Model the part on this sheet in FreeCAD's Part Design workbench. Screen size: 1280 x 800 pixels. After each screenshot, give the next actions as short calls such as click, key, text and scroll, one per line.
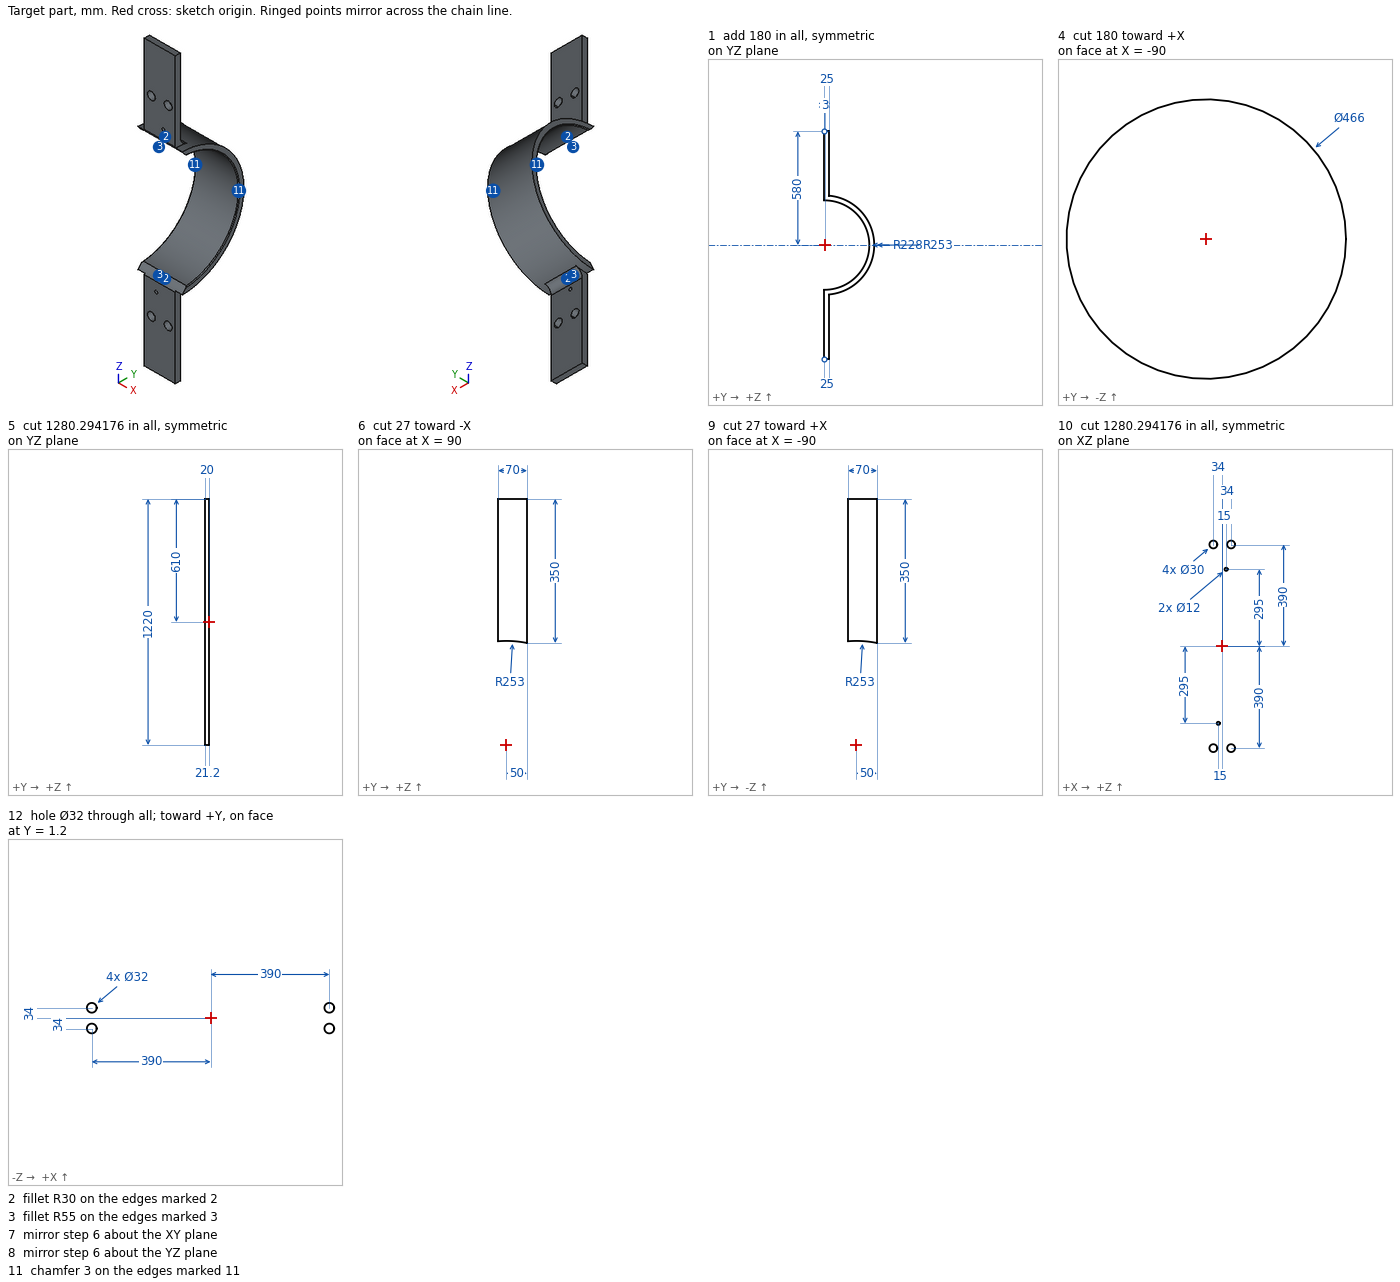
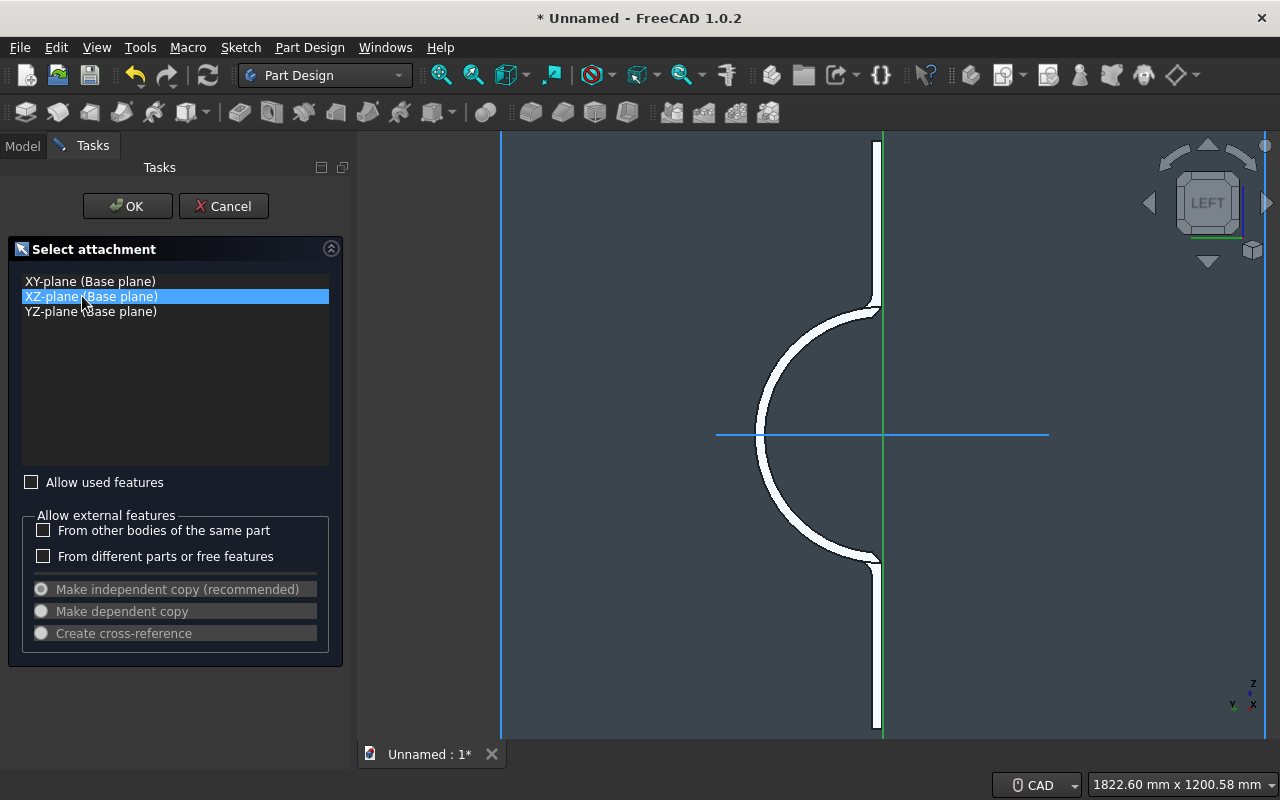
click(128, 206)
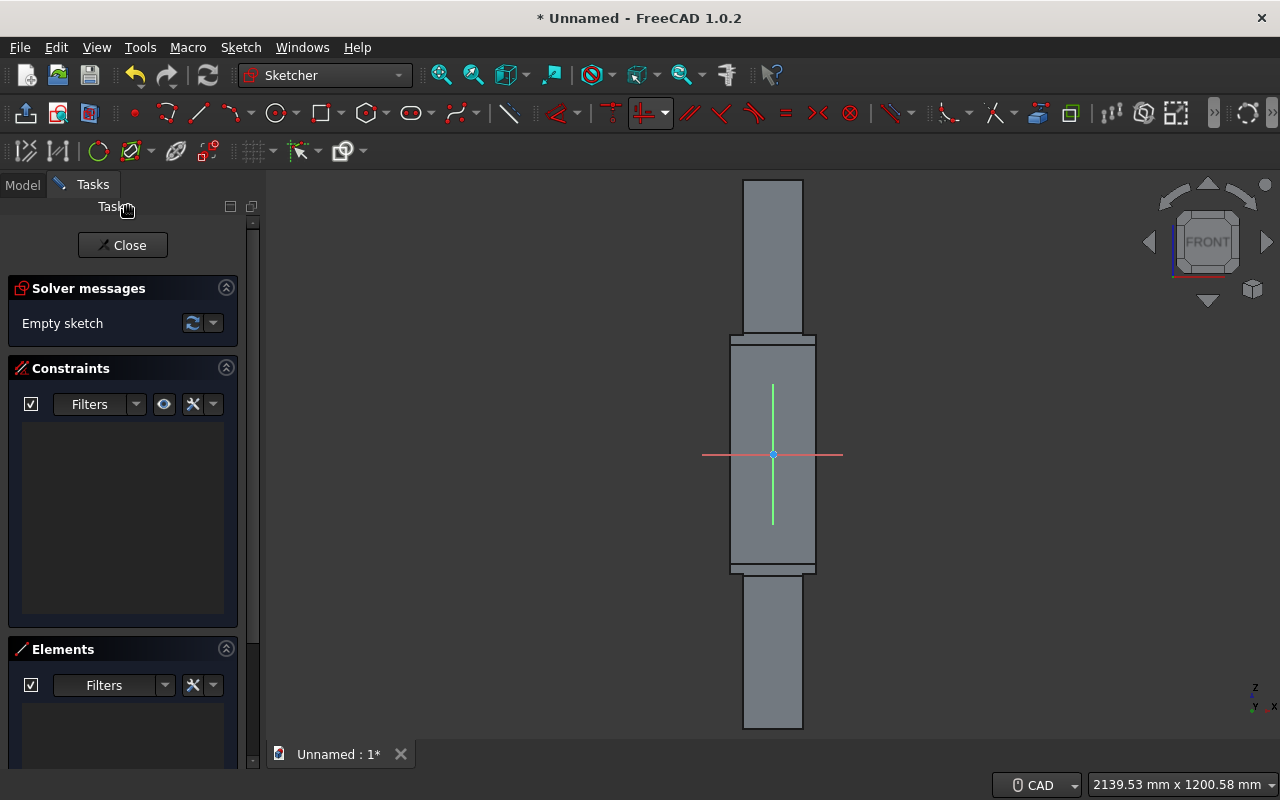
click(276, 114)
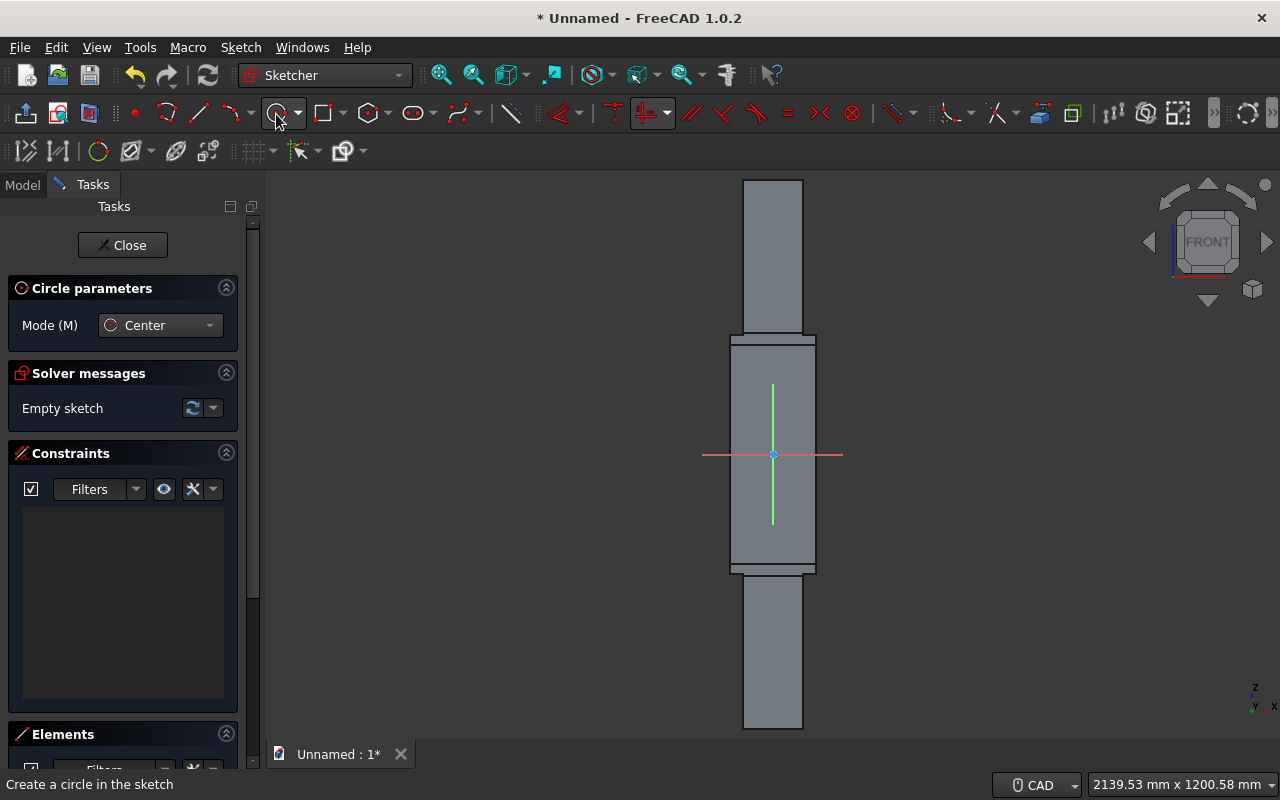
scroll(789, 270, up, 6)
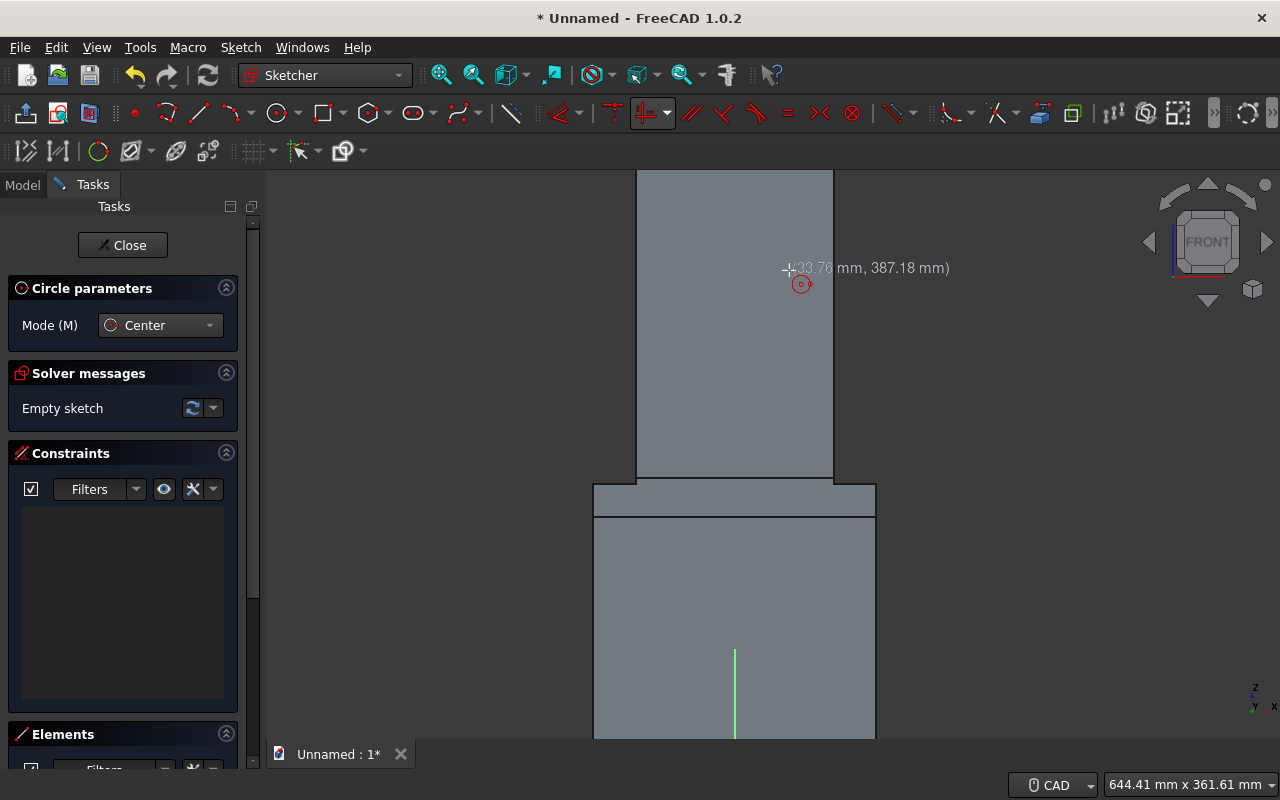
click(788, 268)
move(805, 252)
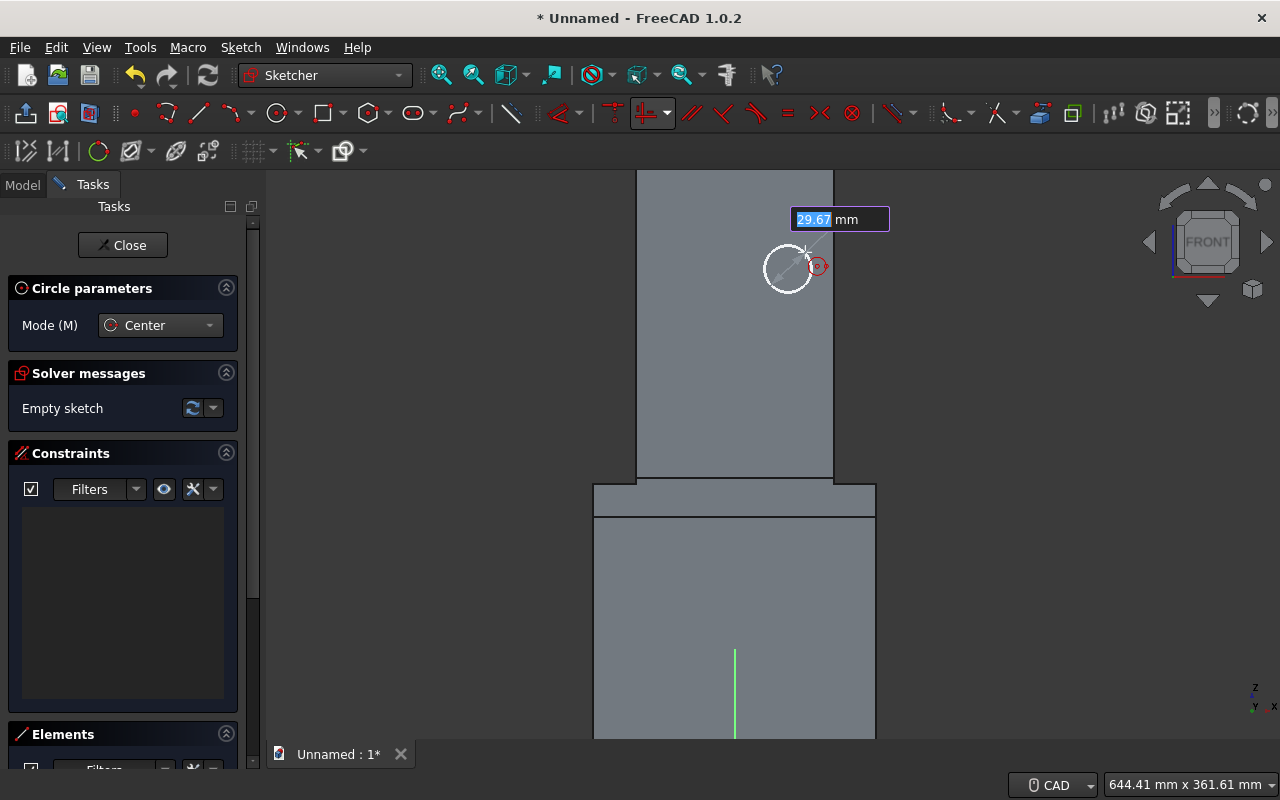
text(30)
key(Return)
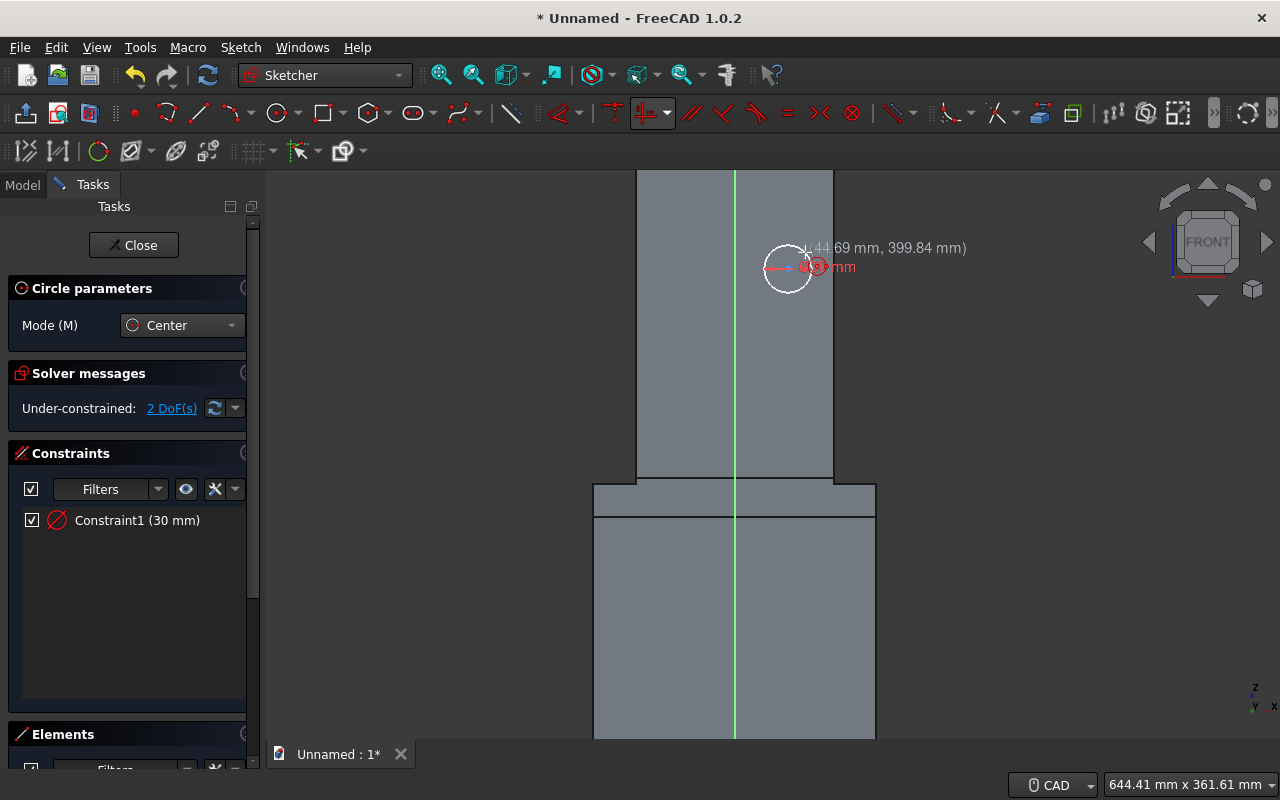
scroll(691, 270, down, 6)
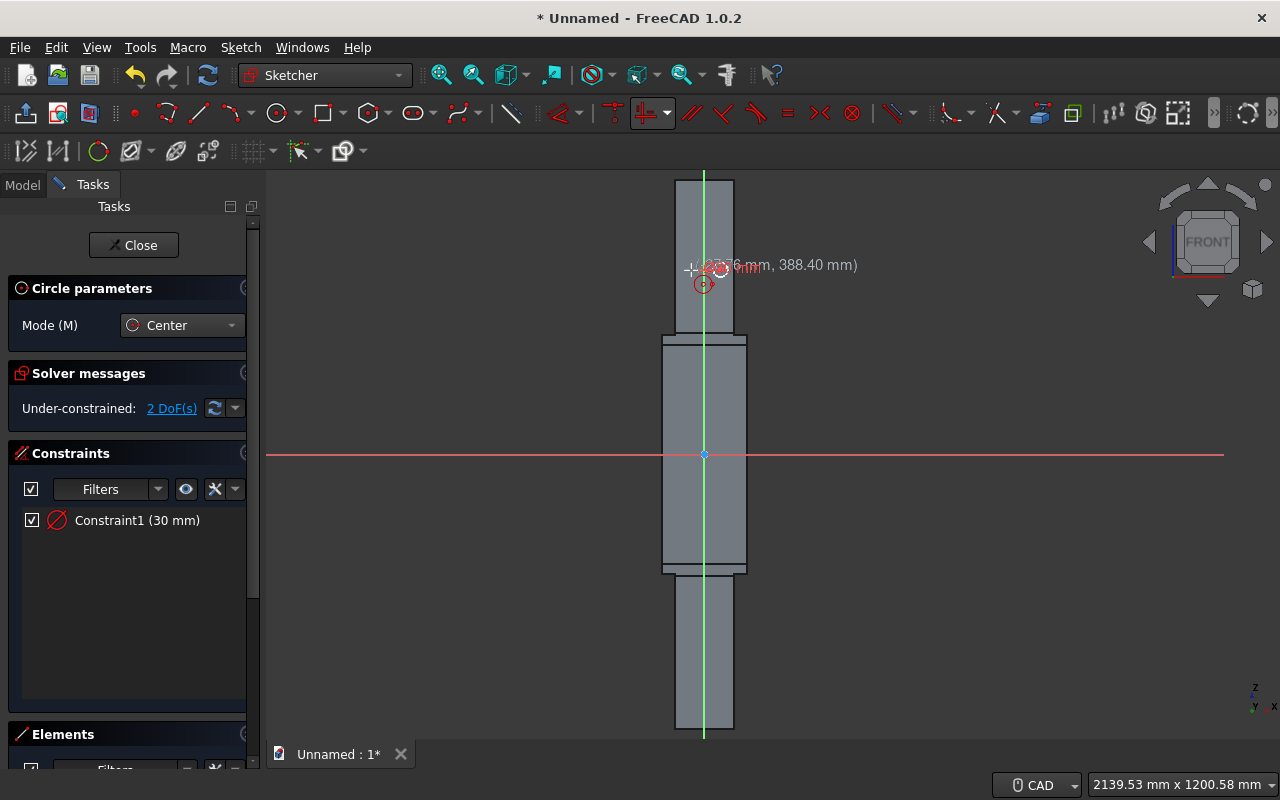
scroll(721, 639, up, 6)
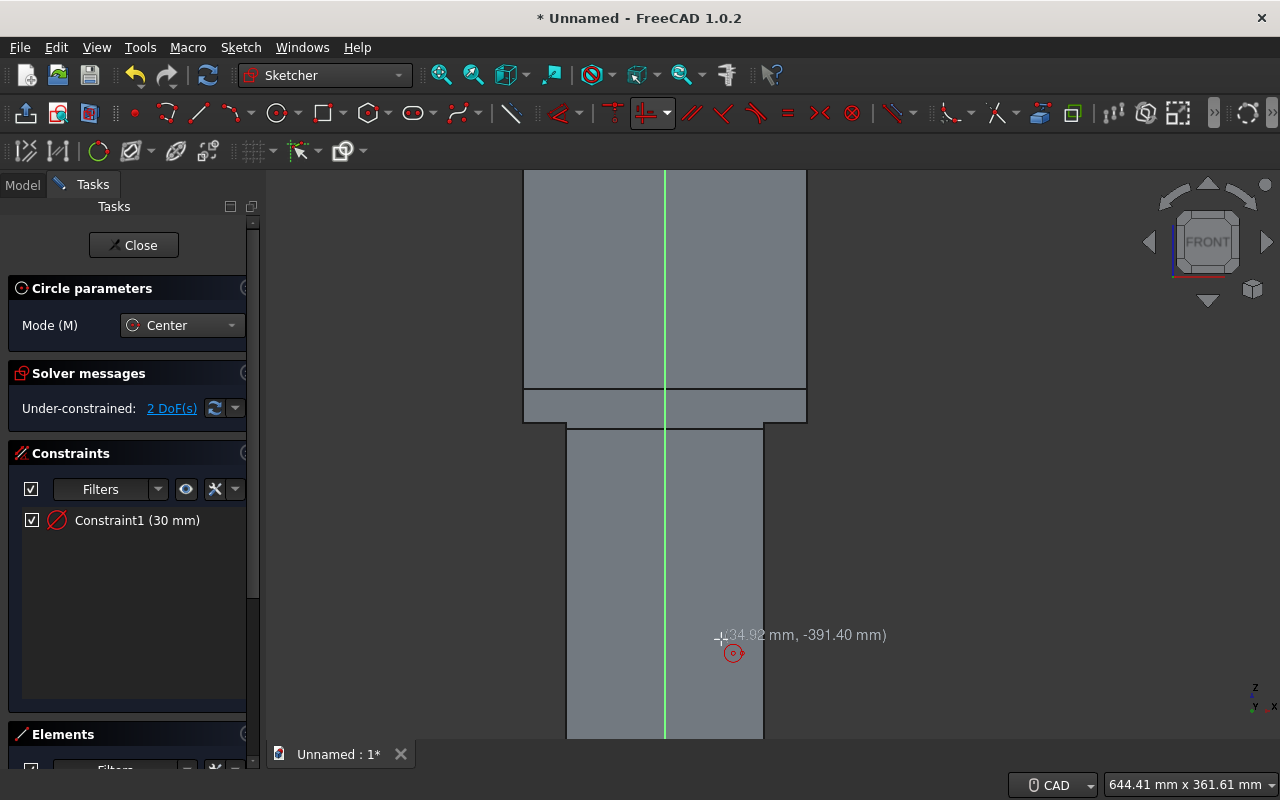
click(719, 638)
move(735, 622)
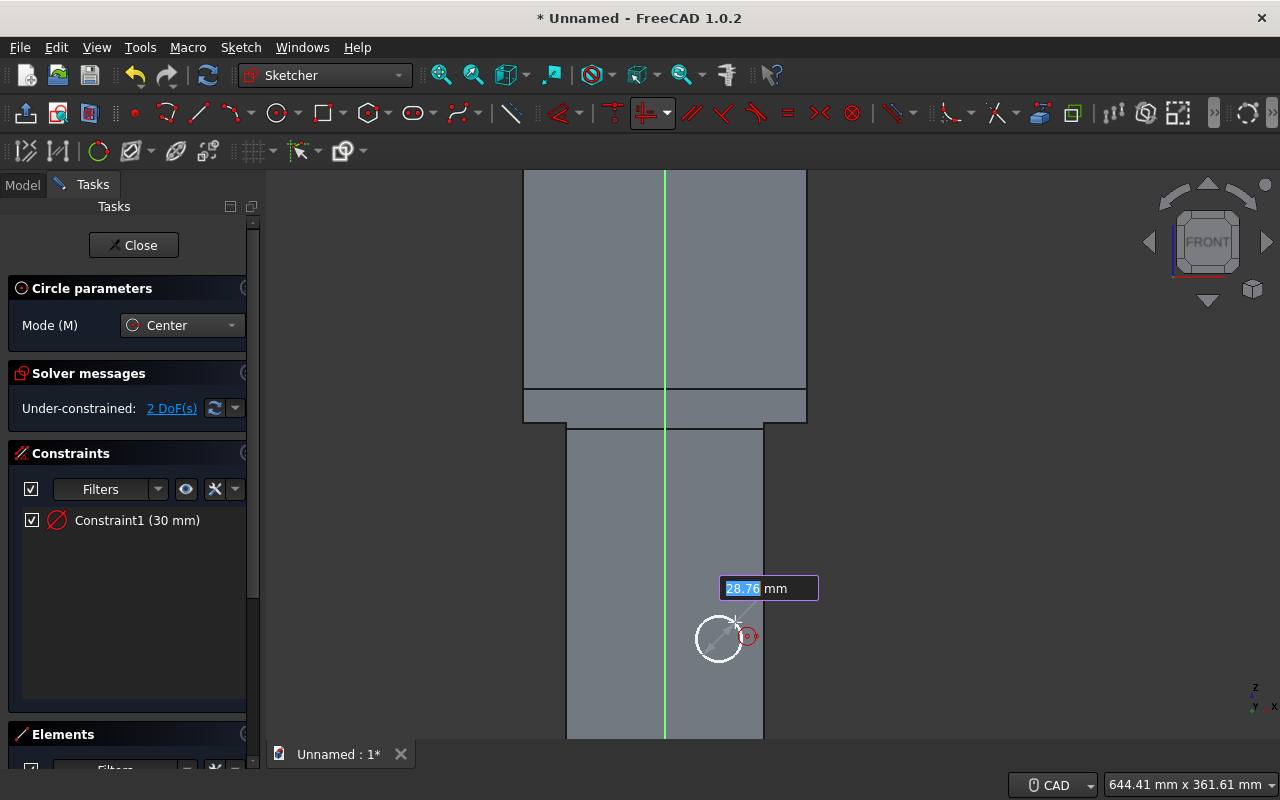
text(30)
key(Return)